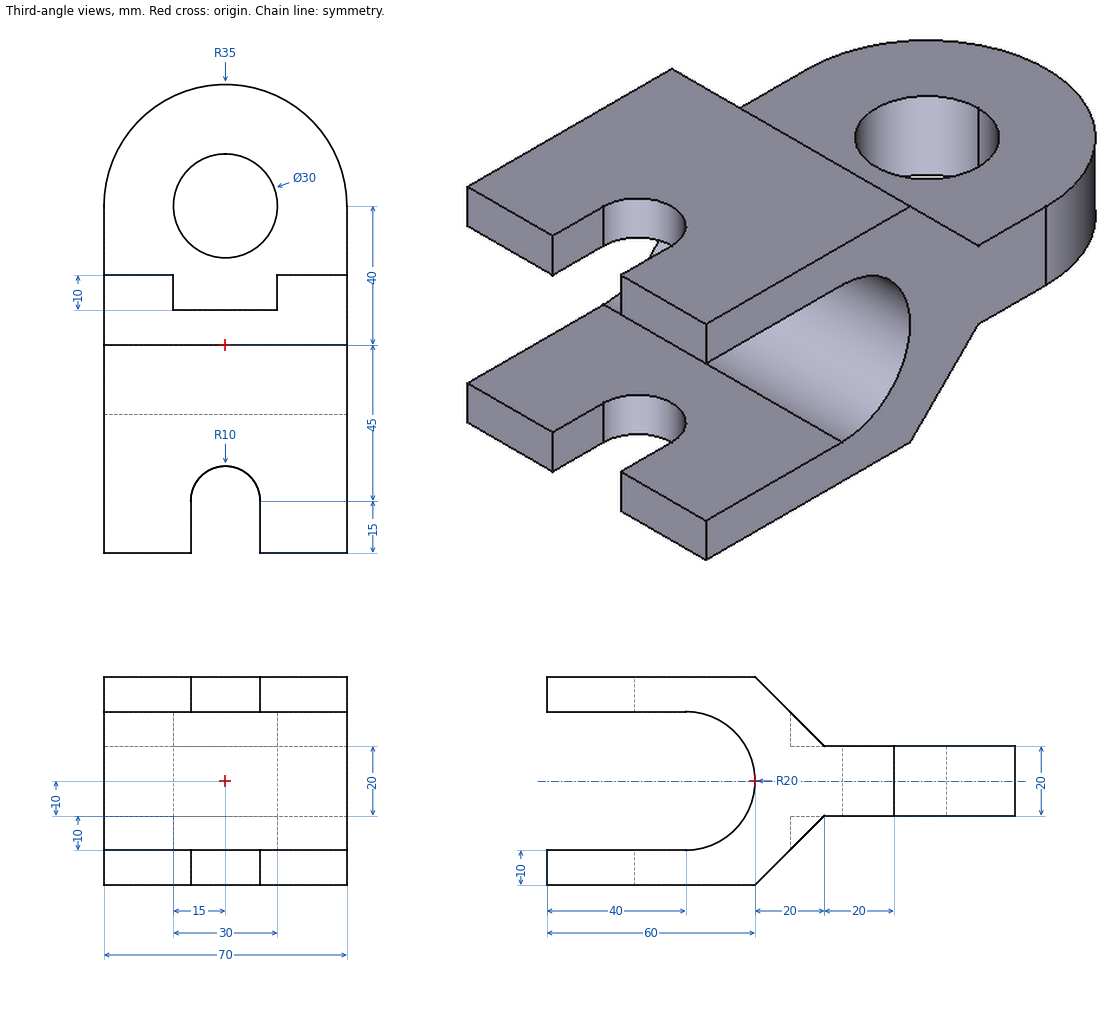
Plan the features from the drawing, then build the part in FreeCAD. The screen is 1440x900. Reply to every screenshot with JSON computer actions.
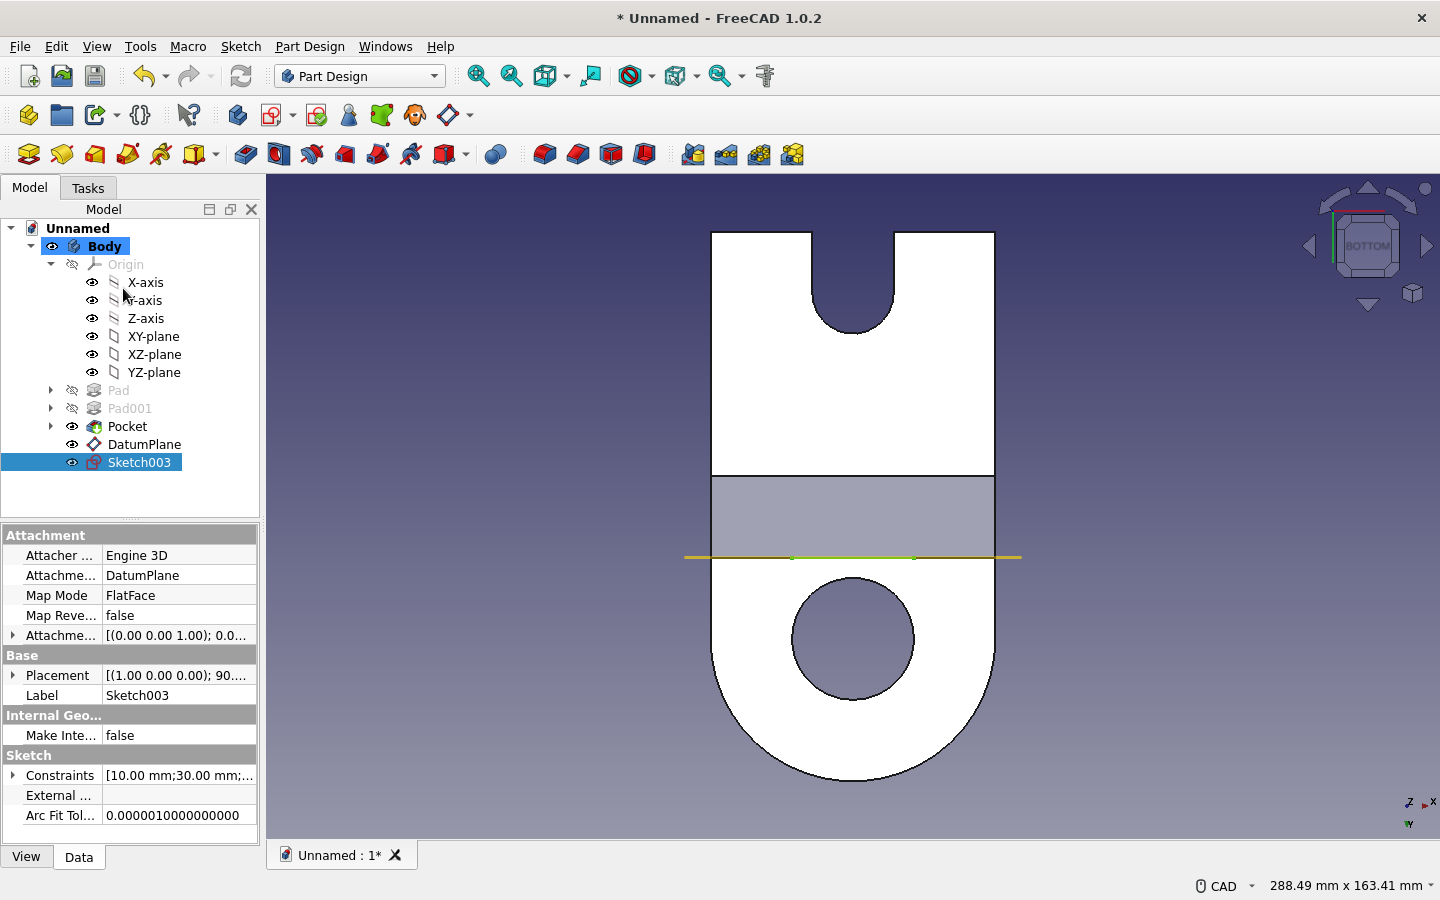
{"action": "left_click", "coordinate": [246, 154]}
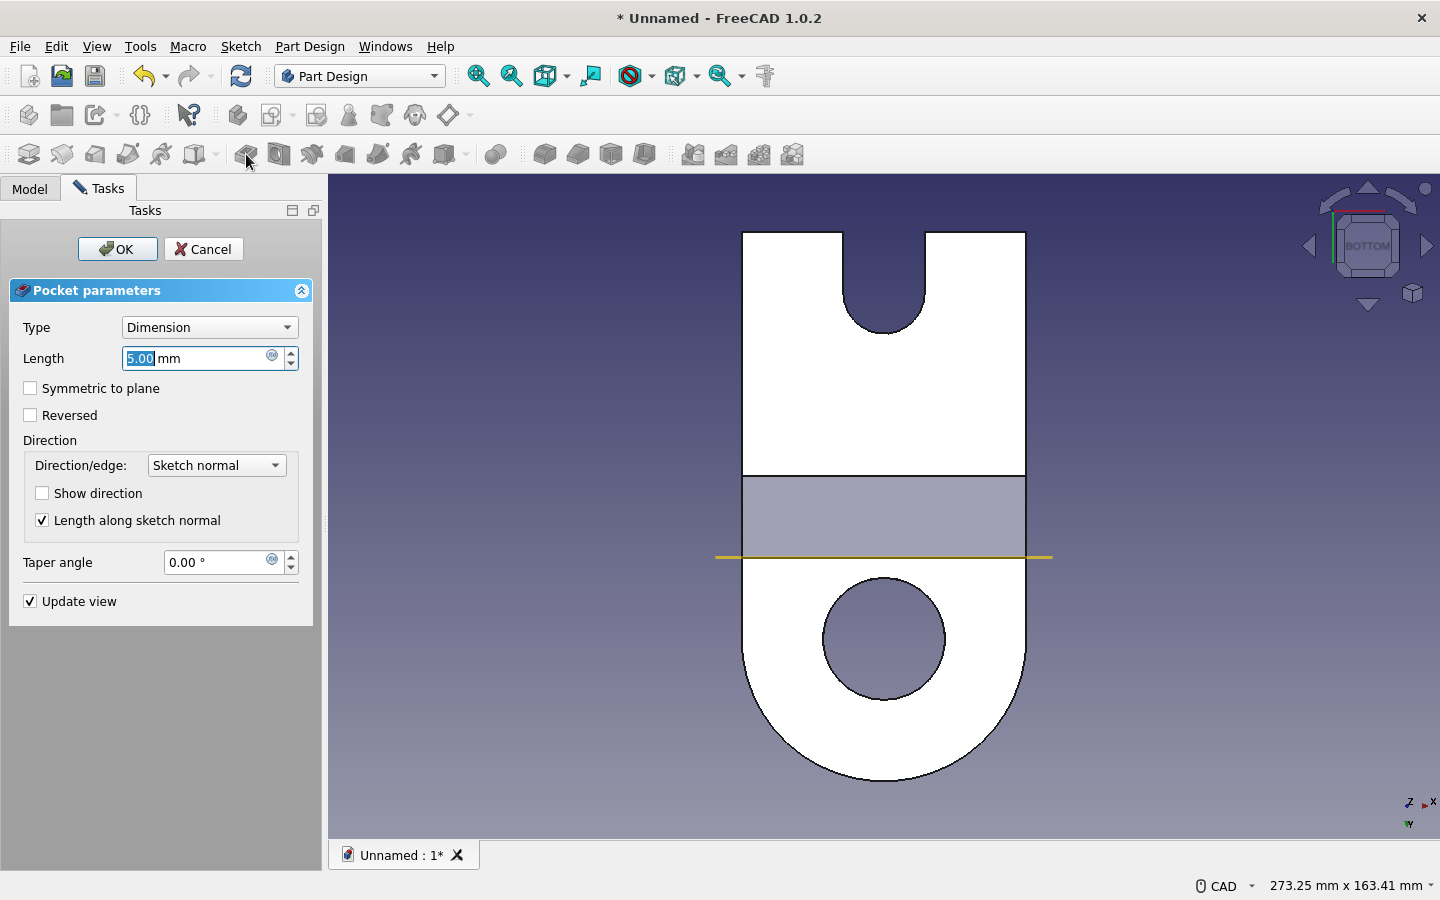
{"action": "type", "text": "10"}
{"action": "key", "text": "Tab"}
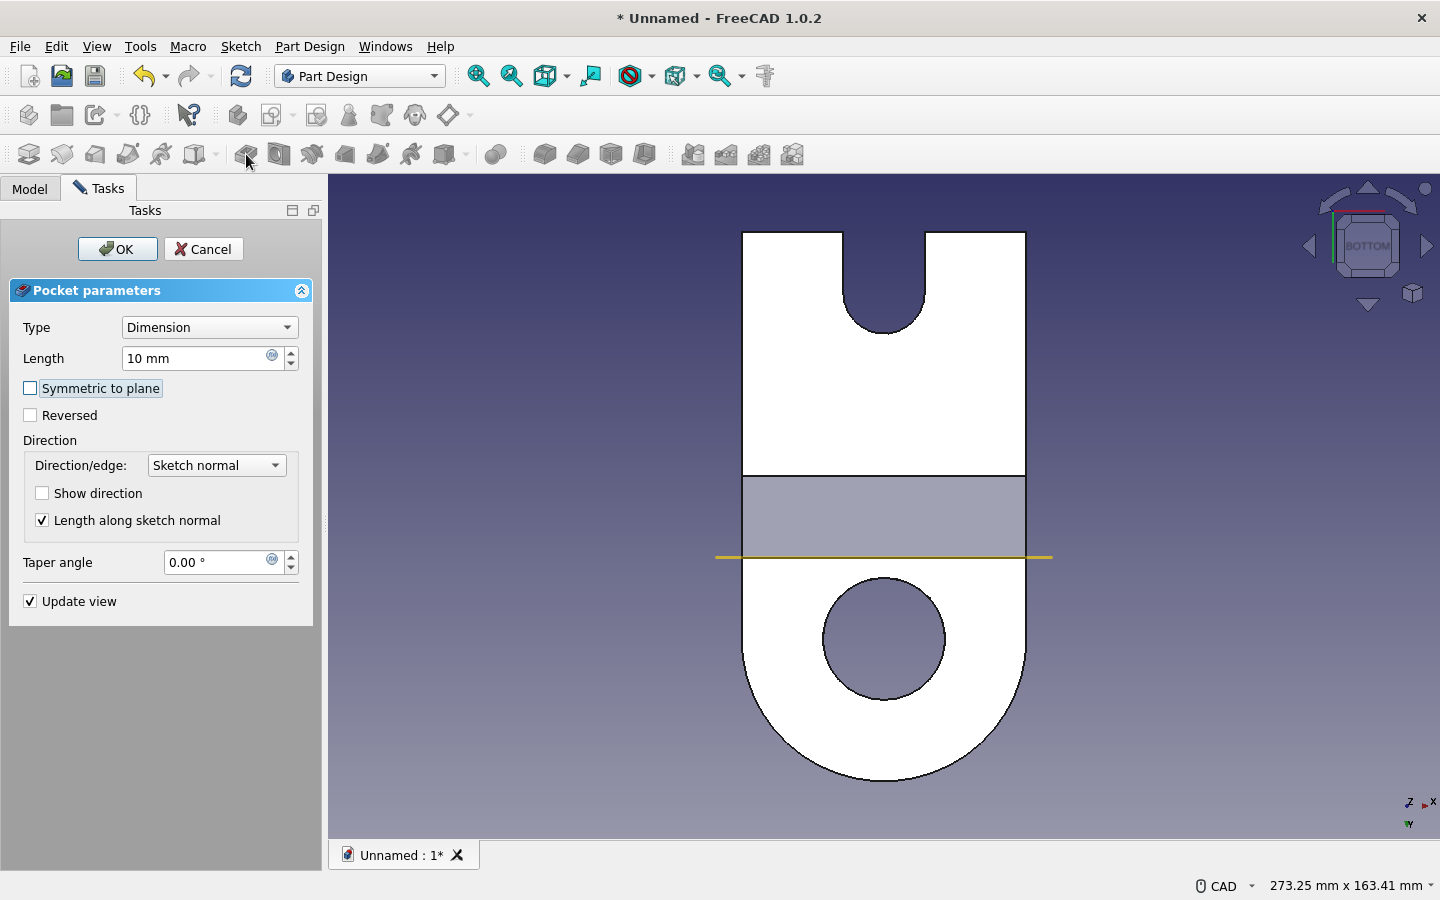
{"action": "left_click", "coordinate": [31, 415]}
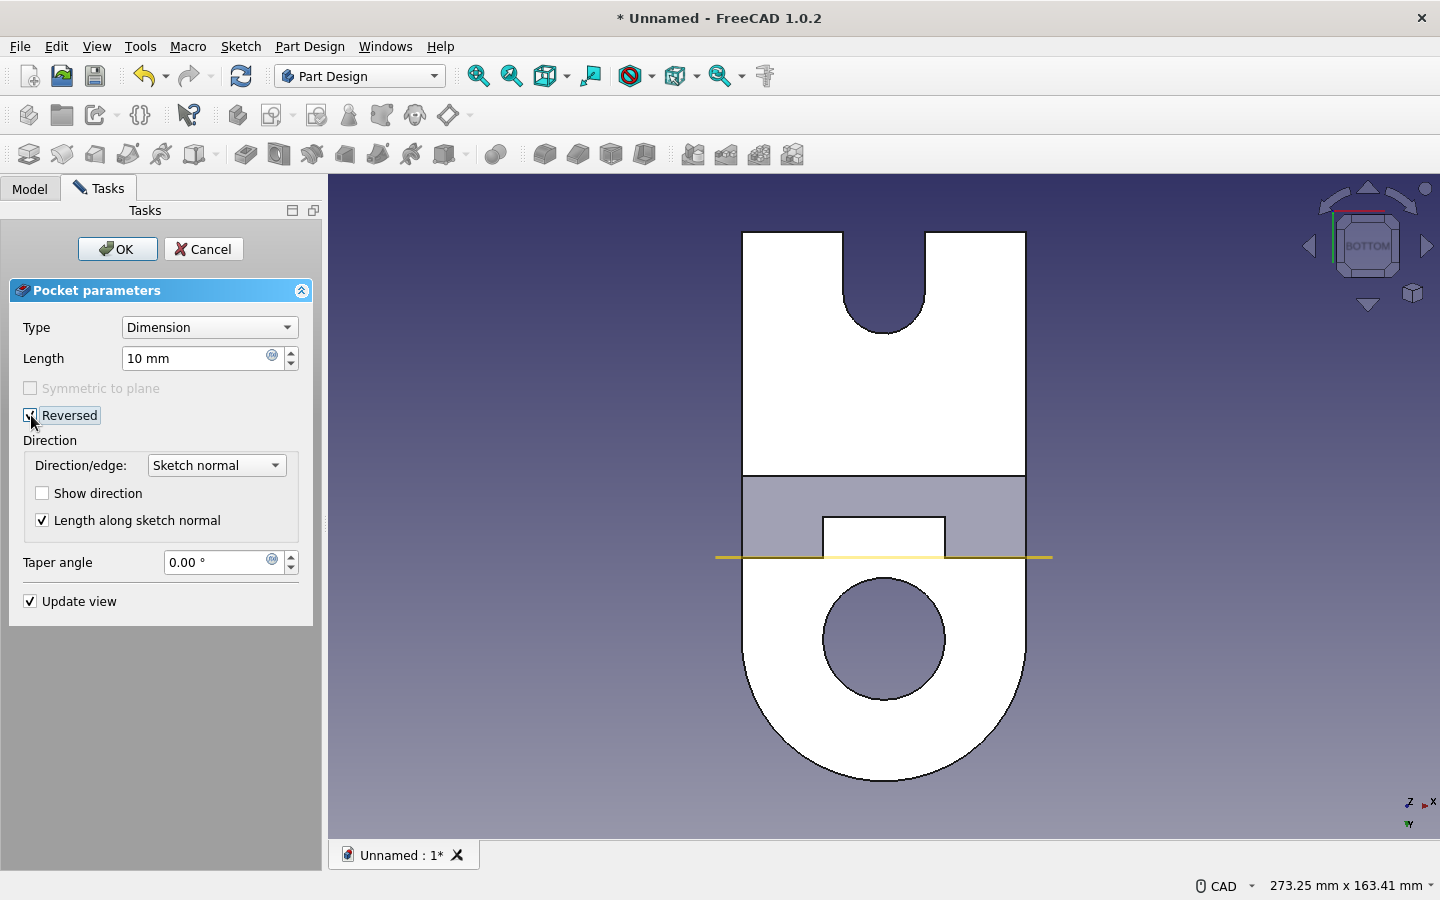
{"action": "left_click", "coordinate": [118, 249]}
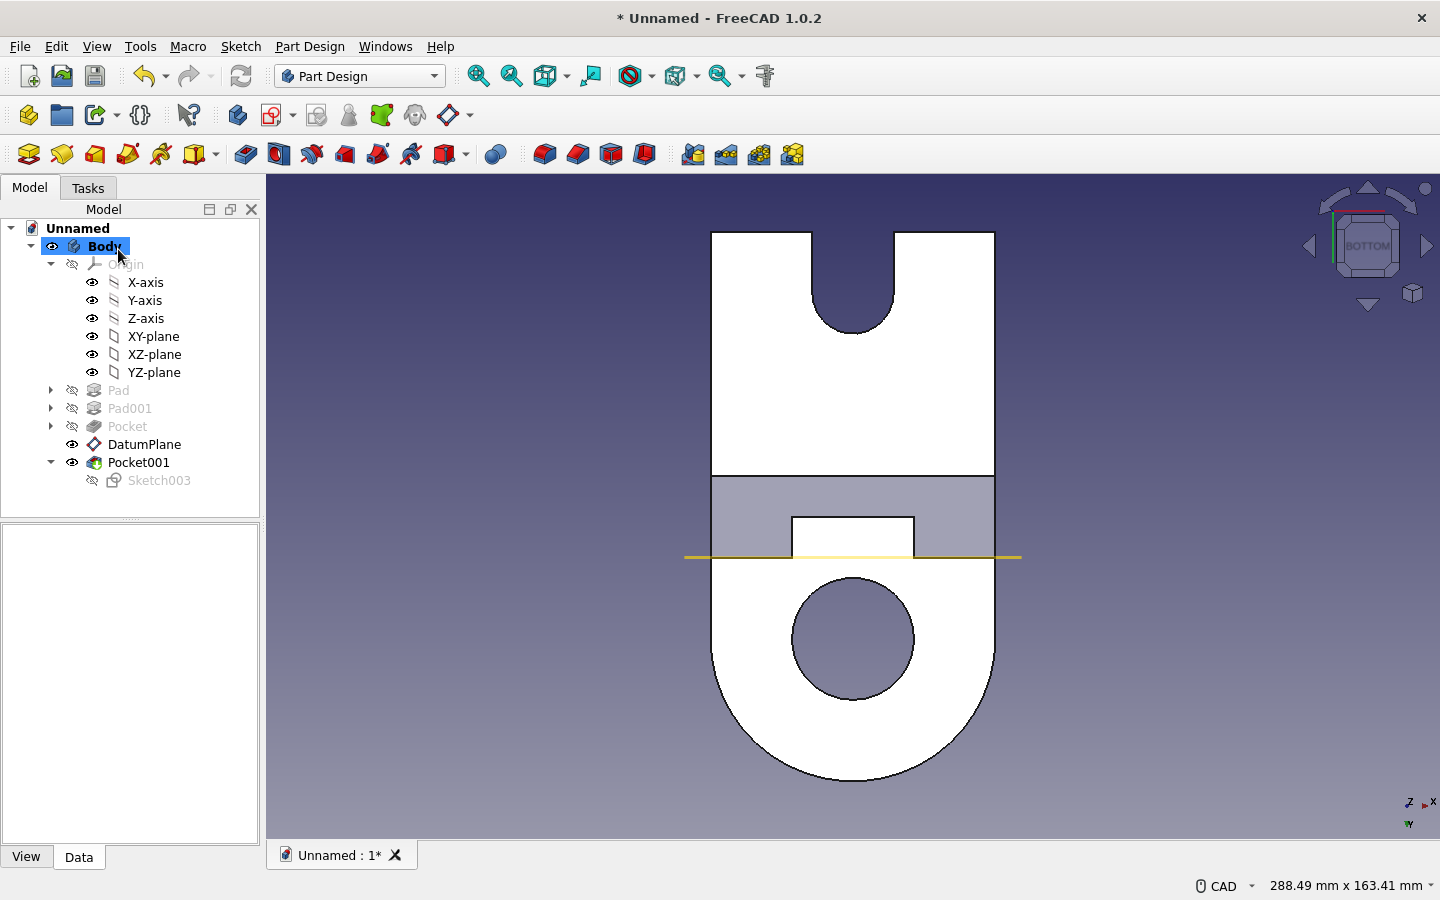
{"action": "left_click", "coordinate": [117, 444]}
{"action": "key", "text": "space"}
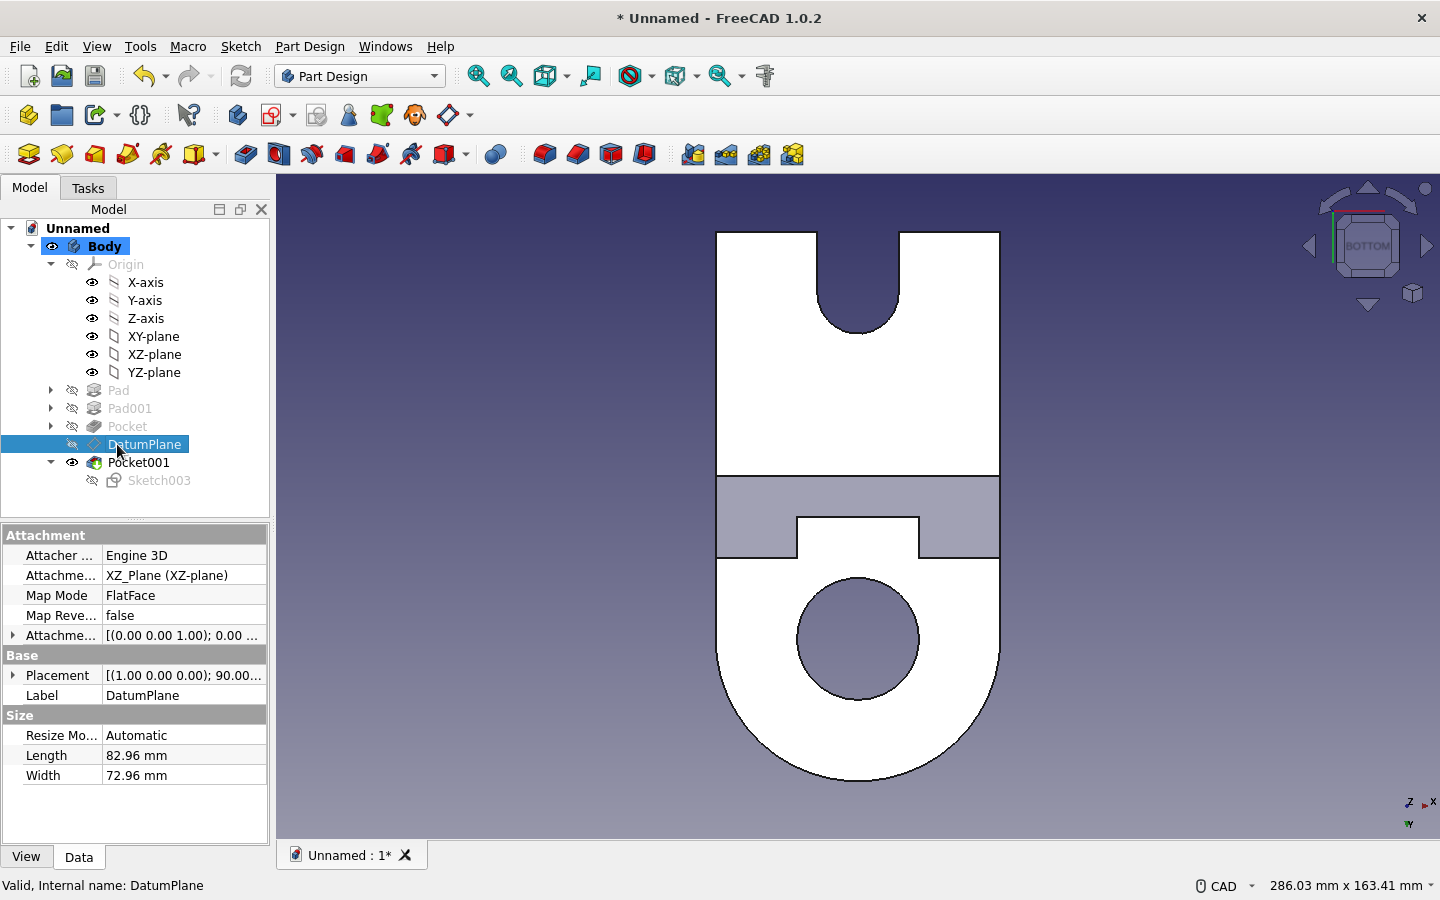
{"action": "left_click", "coordinate": [117, 462]}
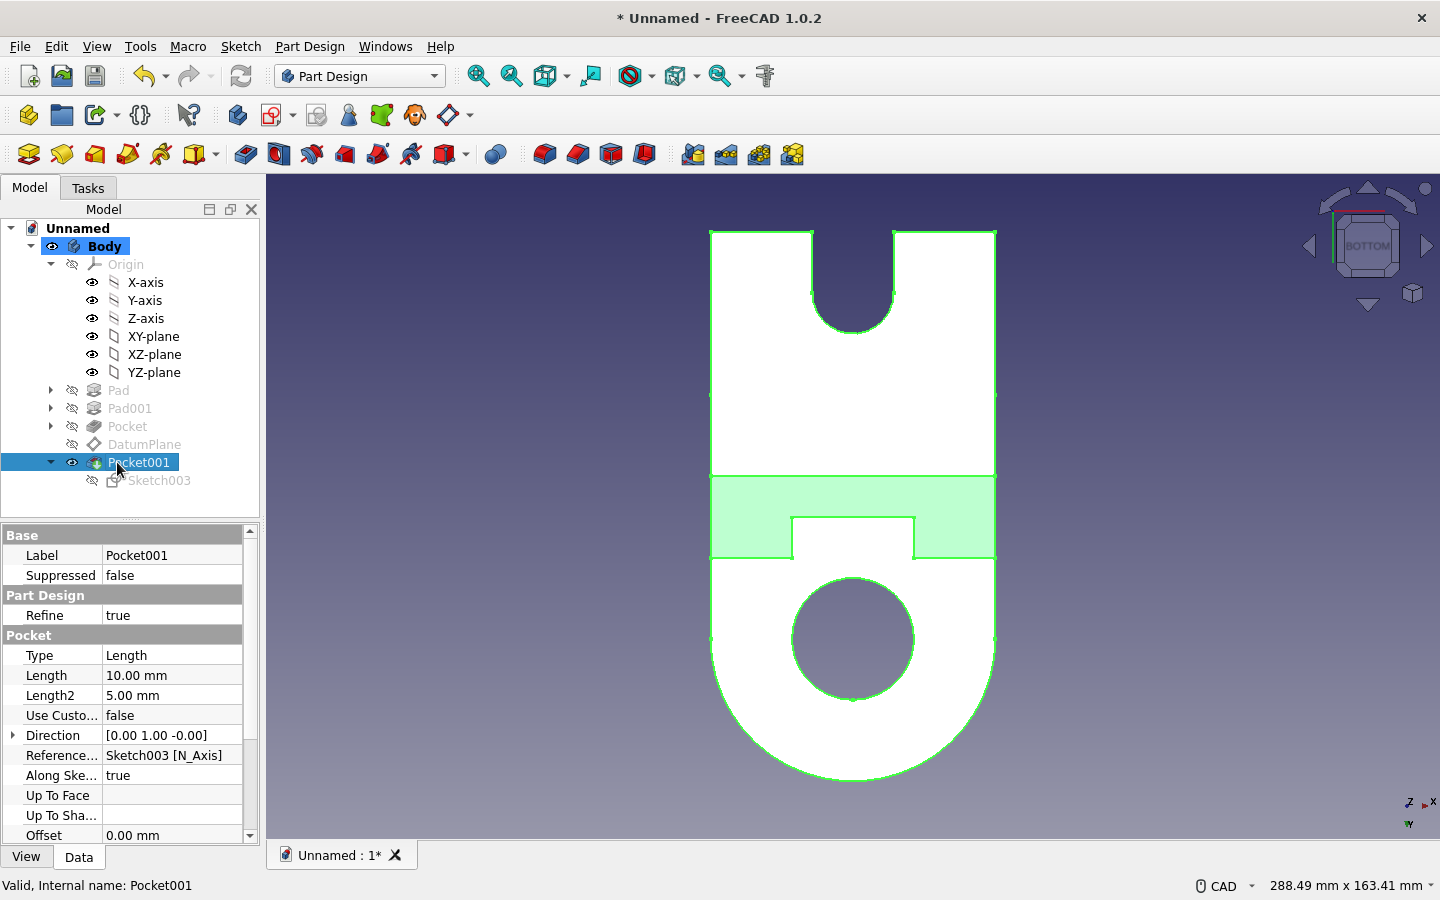
{"action": "left_click", "coordinate": [693, 154]}